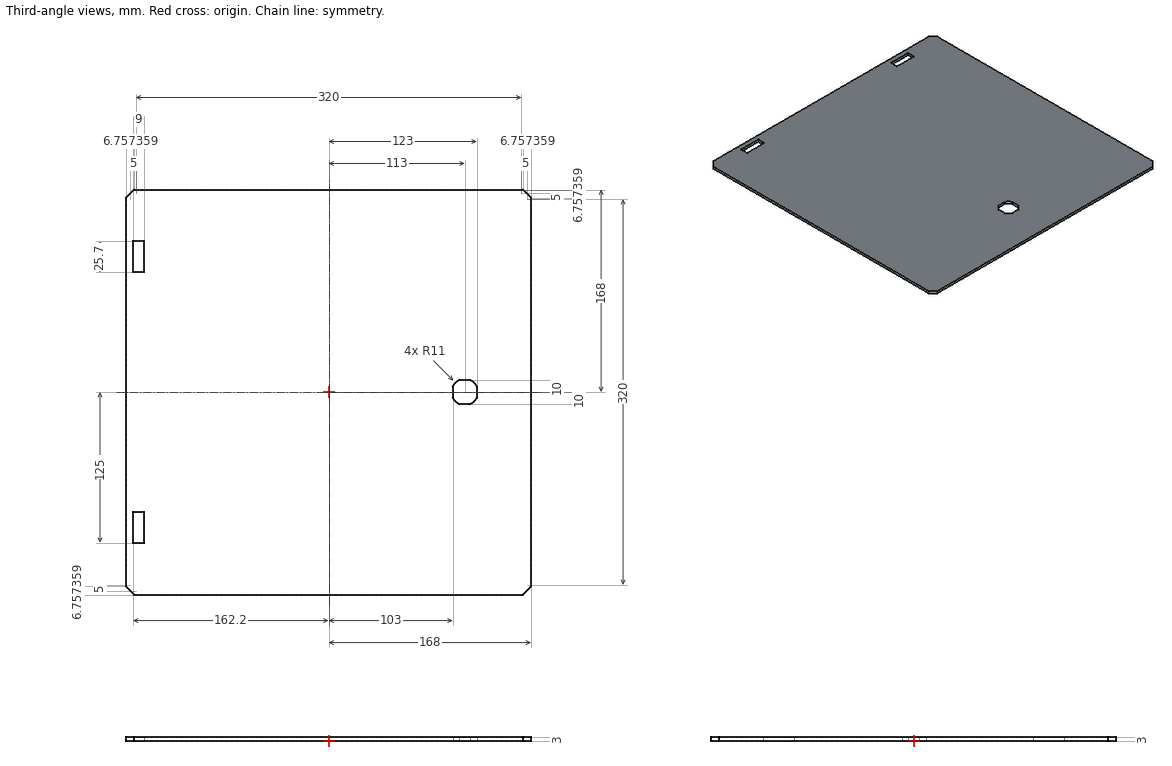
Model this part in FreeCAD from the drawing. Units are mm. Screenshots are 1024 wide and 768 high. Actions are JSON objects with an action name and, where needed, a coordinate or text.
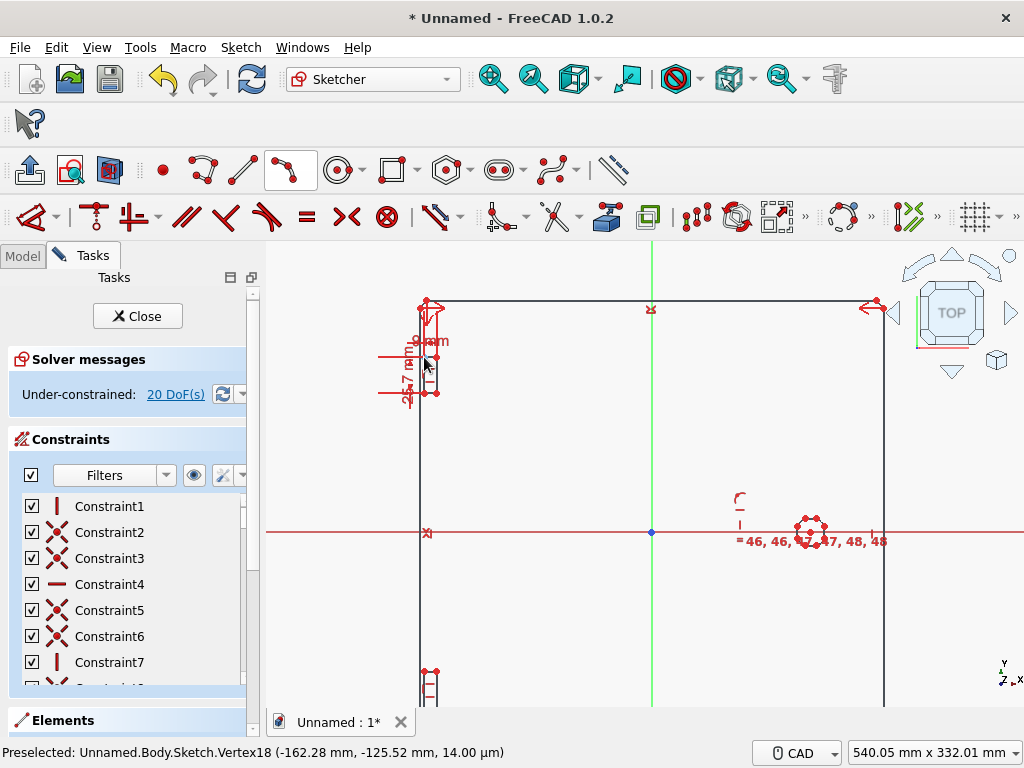
{"action": "left_click", "coordinate": [424, 357]}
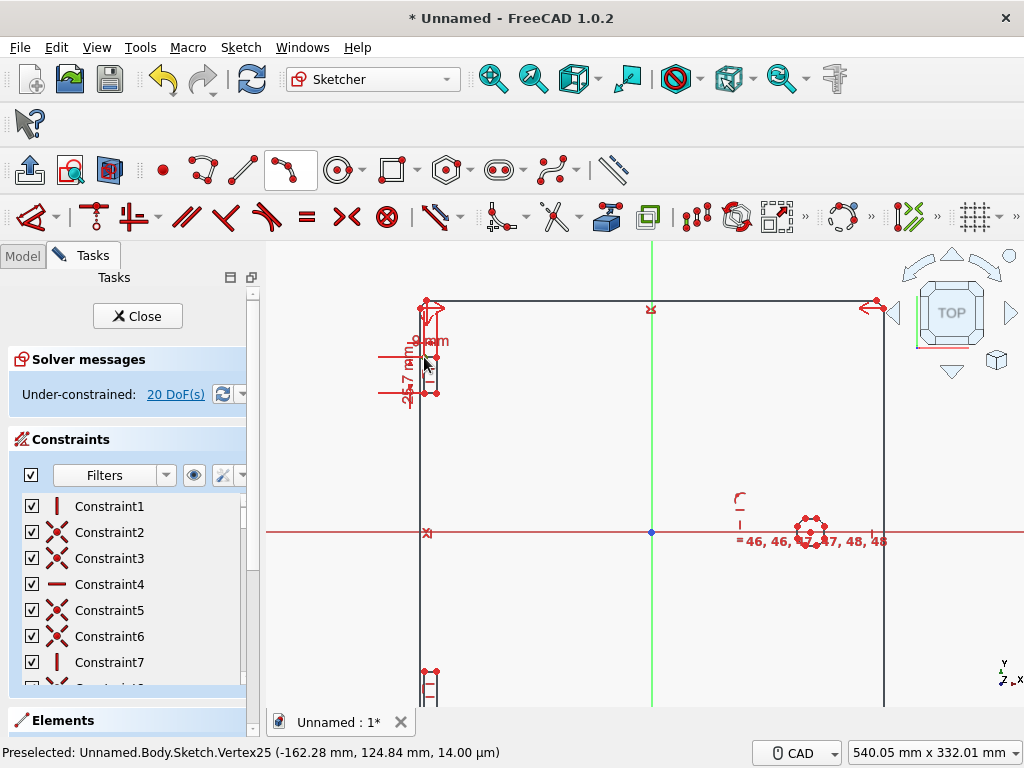
{"action": "left_click", "coordinate": [334, 532]}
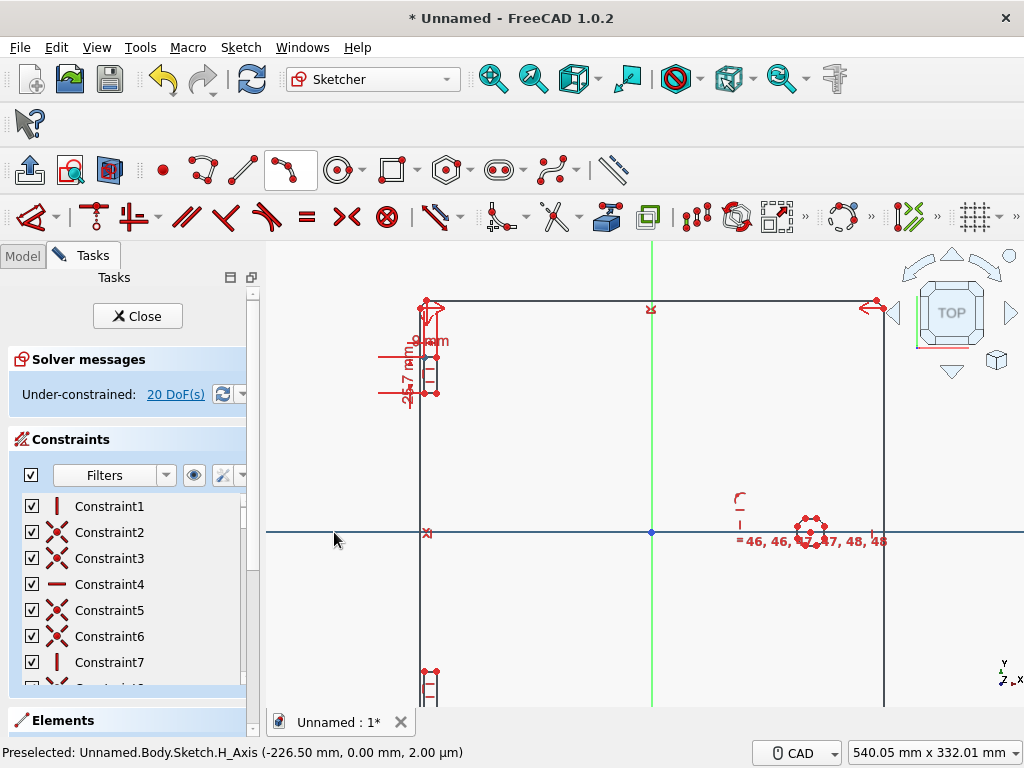
{"action": "left_click", "coordinate": [348, 218]}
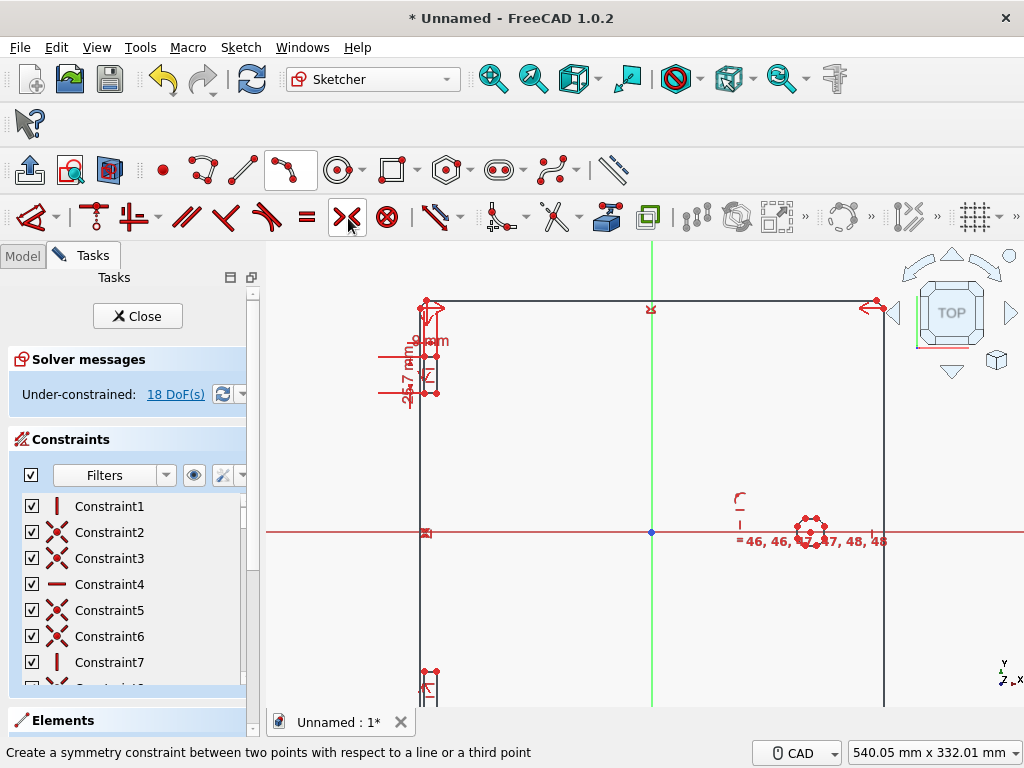
{"action": "left_click", "coordinate": [437, 672]}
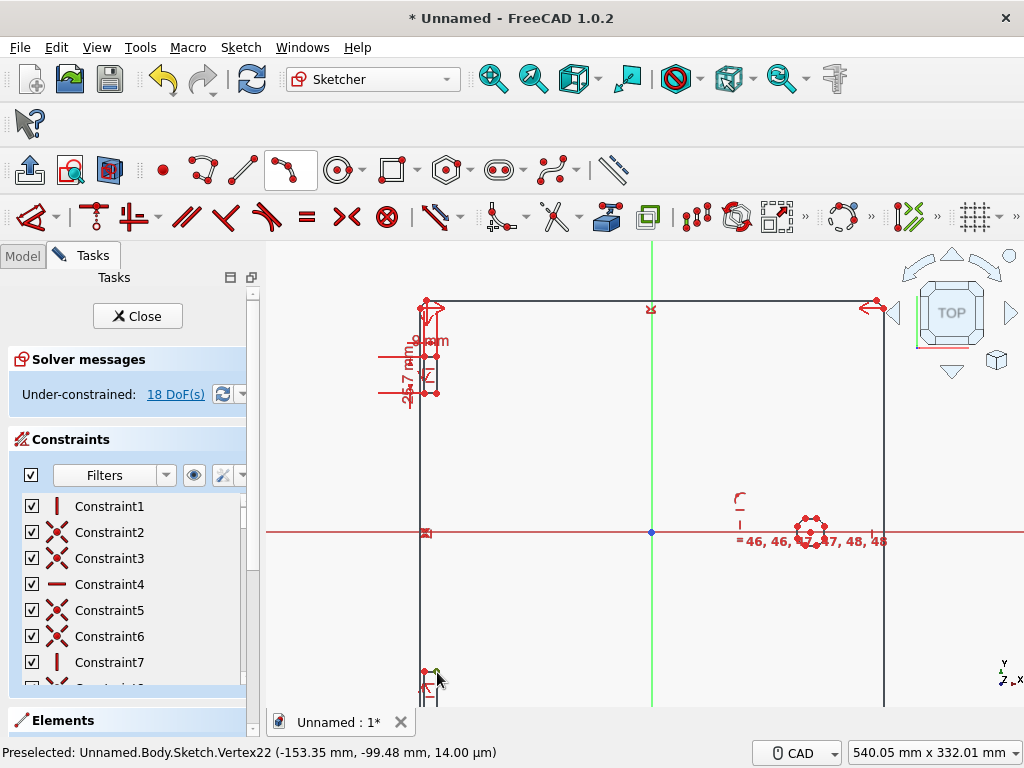
{"action": "left_click", "coordinate": [437, 393]}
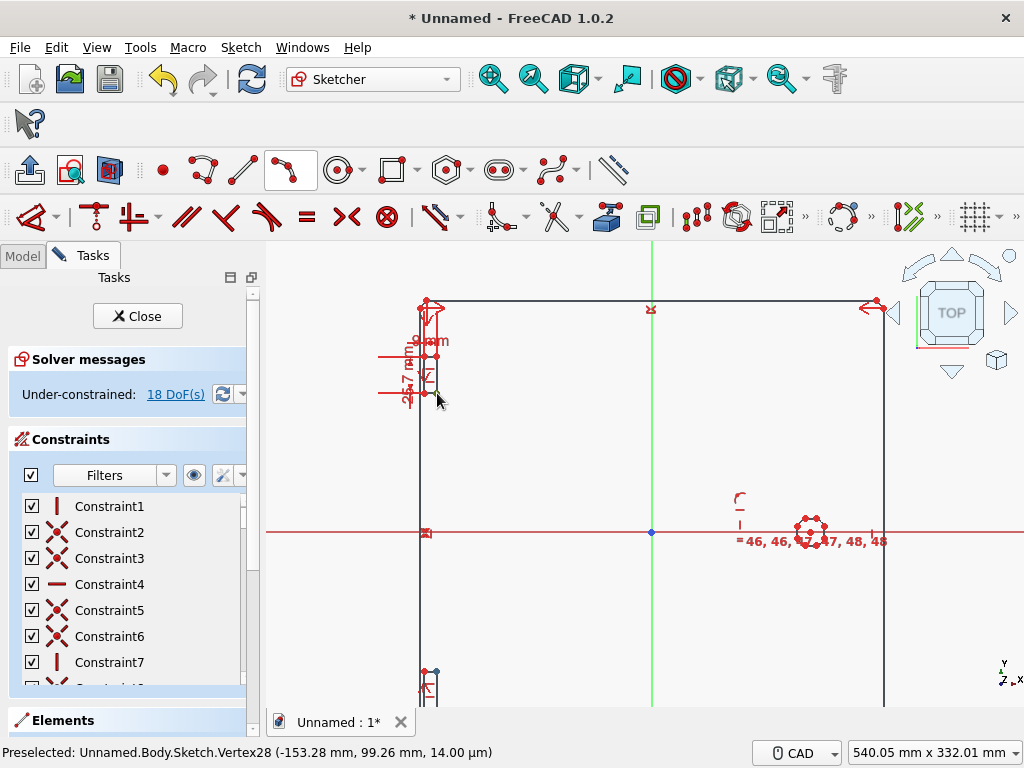
{"action": "left_click", "coordinate": [334, 532]}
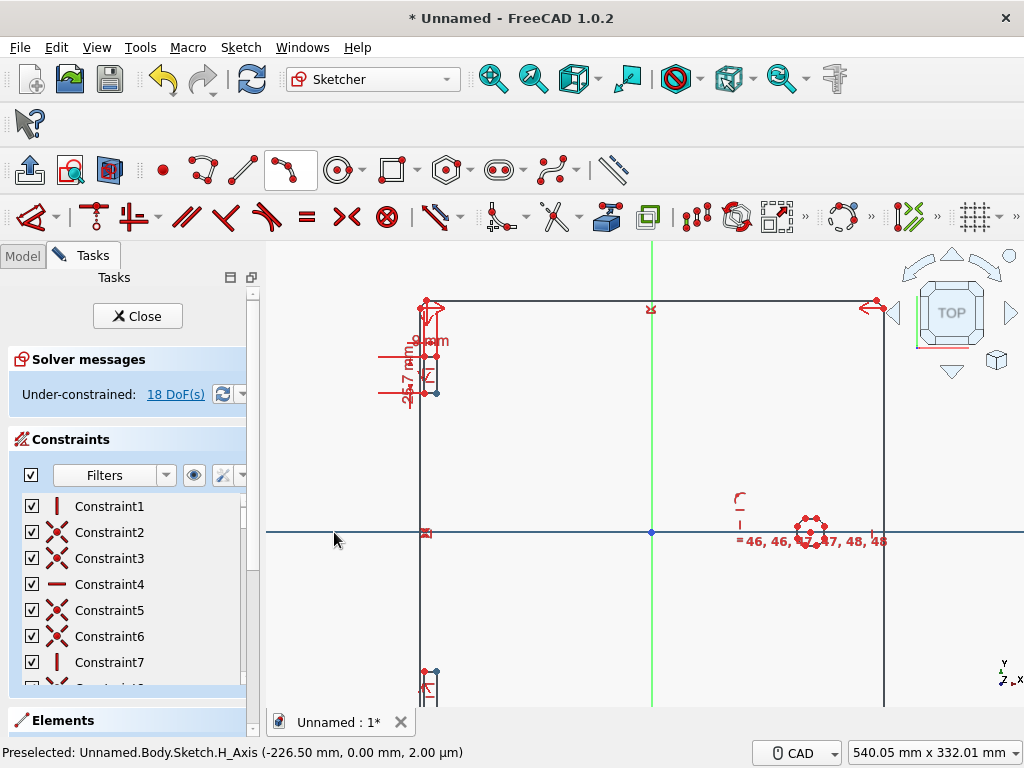
{"action": "left_click", "coordinate": [348, 218]}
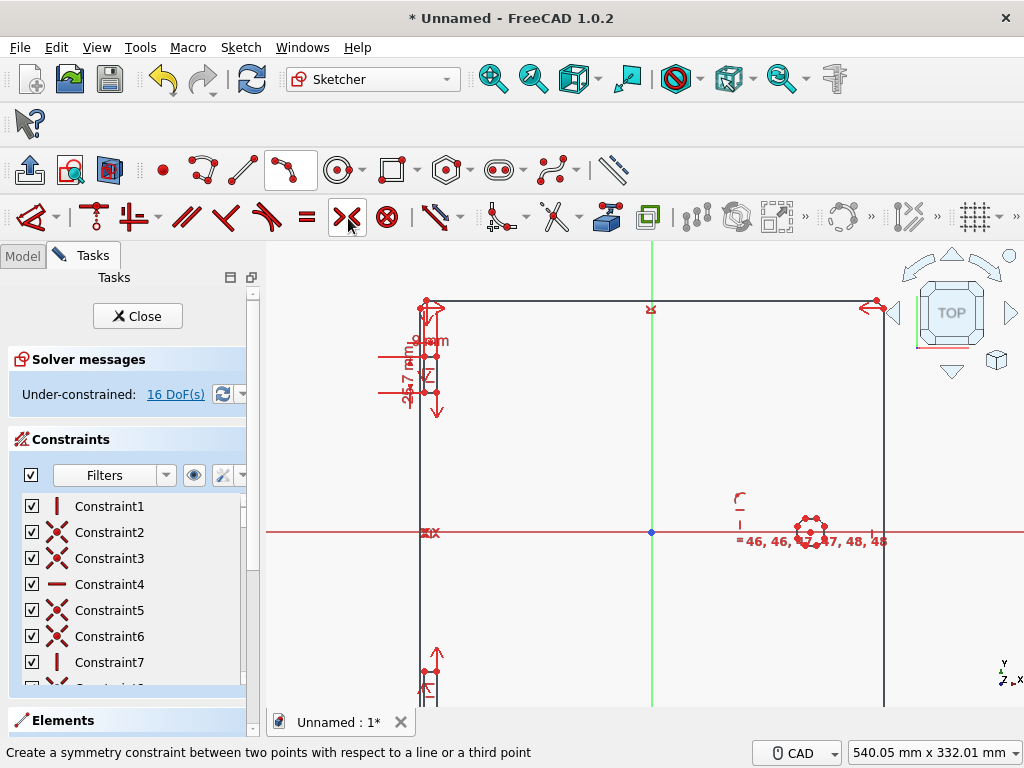
{"action": "left_click", "coordinate": [32, 218]}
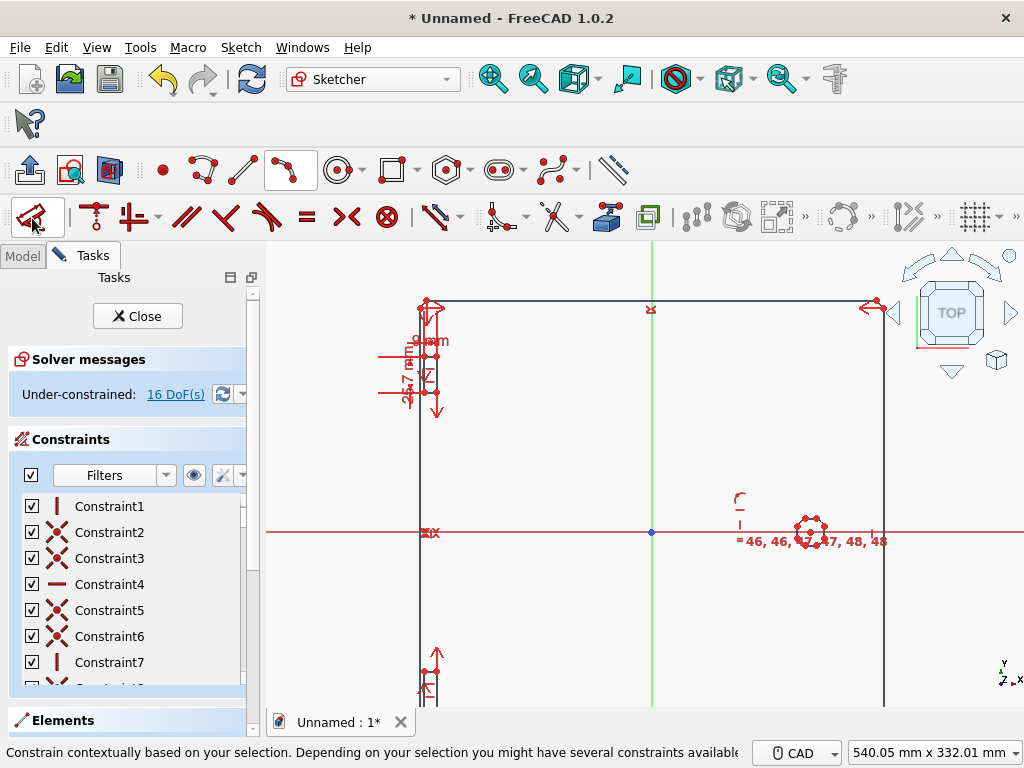
{"action": "scroll", "coordinate": [821, 522], "scroll_direction": "up", "scroll_amount": 5}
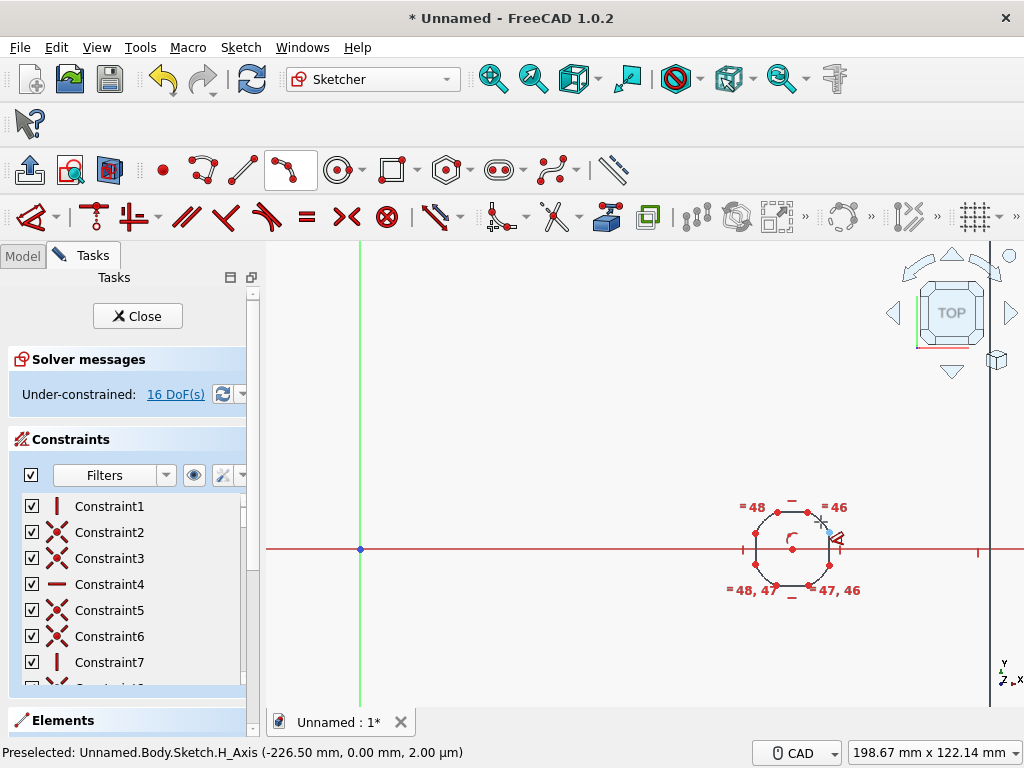
{"action": "left_click", "coordinate": [820, 520]}
{"action": "left_click", "coordinate": [842, 497]}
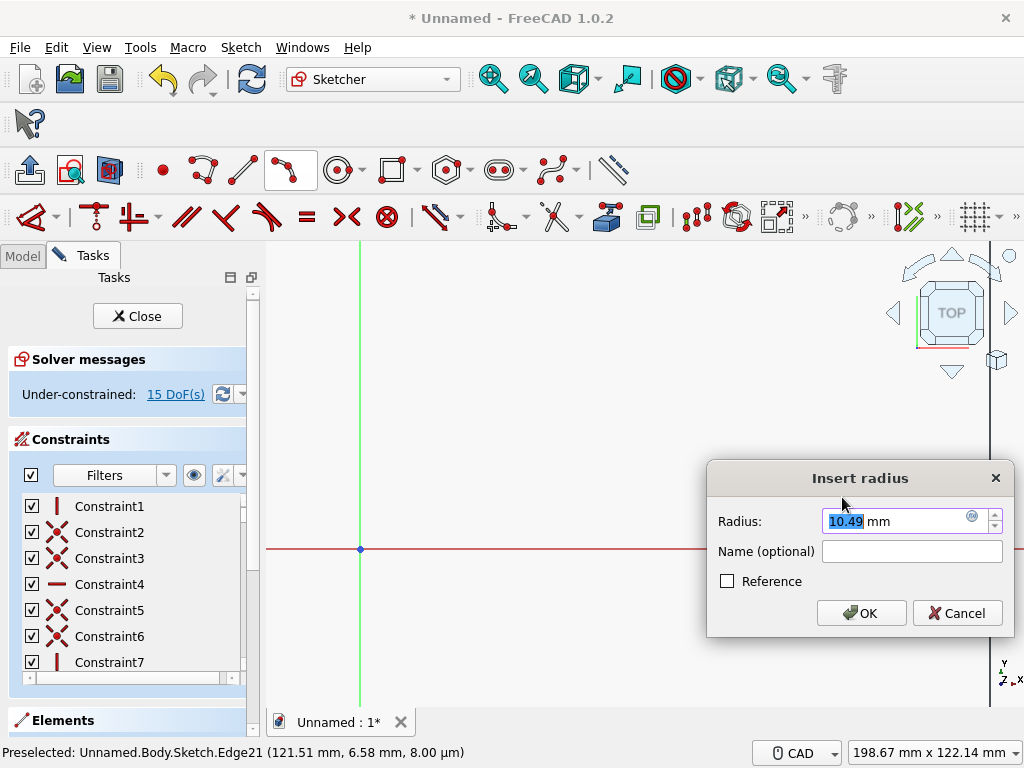
{"action": "type", "text": "11"}
{"action": "key", "text": "Return"}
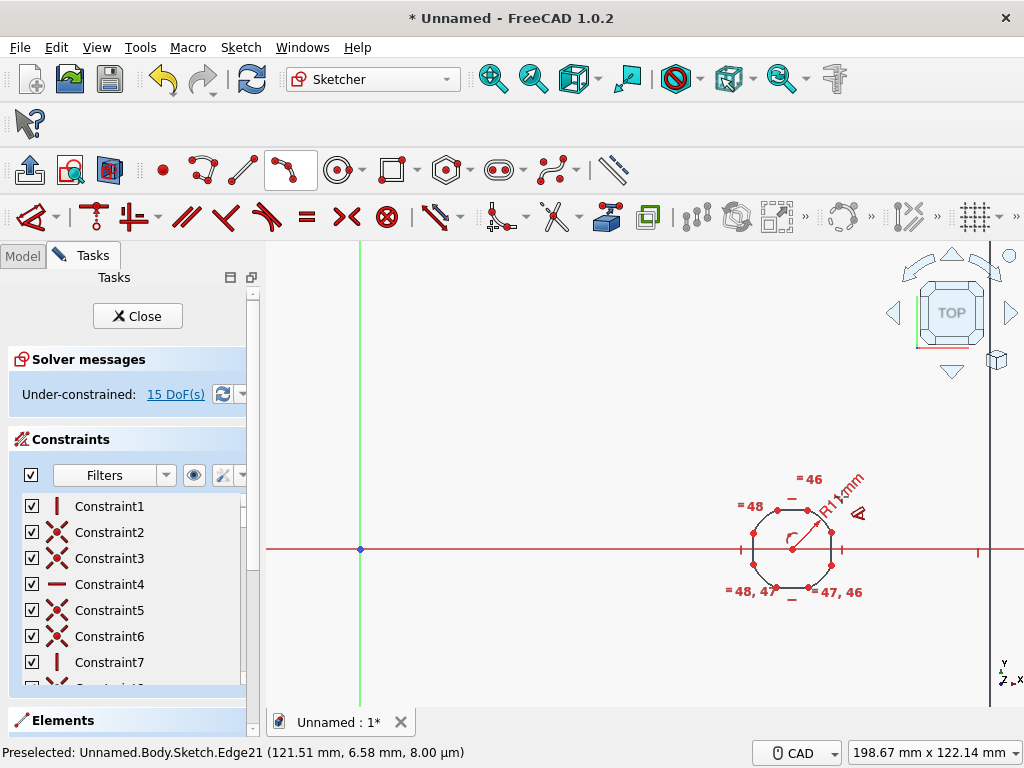
{"action": "scroll", "coordinate": [647, 449], "scroll_direction": "down", "scroll_amount": 7}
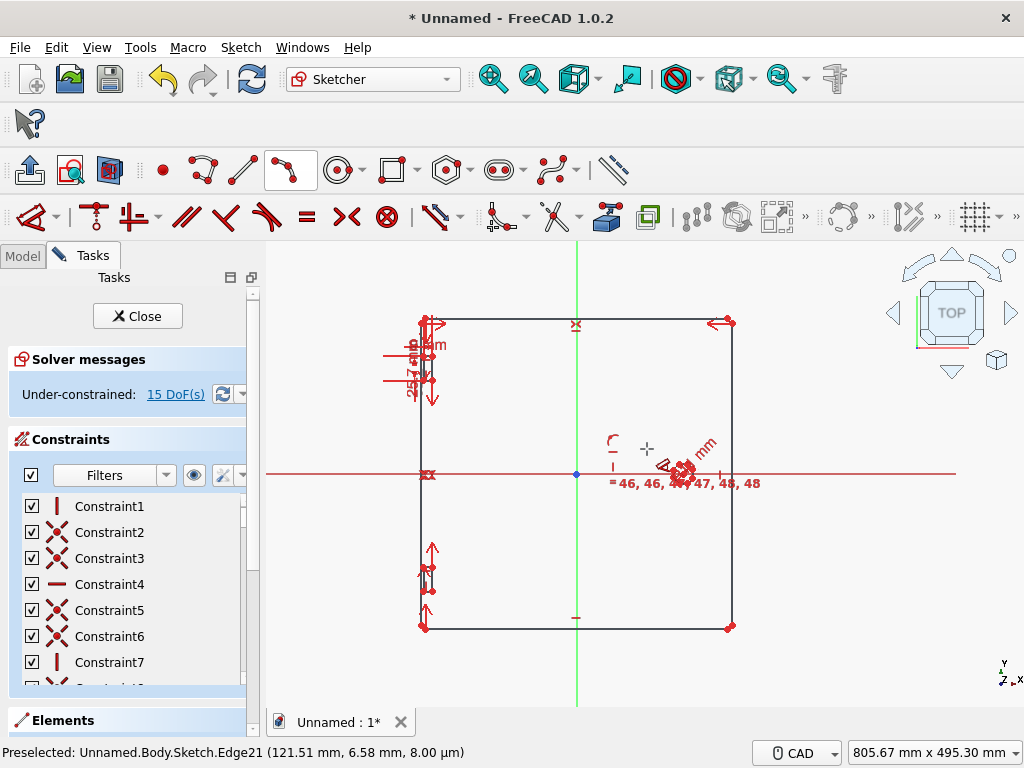
{"action": "scroll", "coordinate": [730, 322], "scroll_direction": "up", "scroll_amount": 11}